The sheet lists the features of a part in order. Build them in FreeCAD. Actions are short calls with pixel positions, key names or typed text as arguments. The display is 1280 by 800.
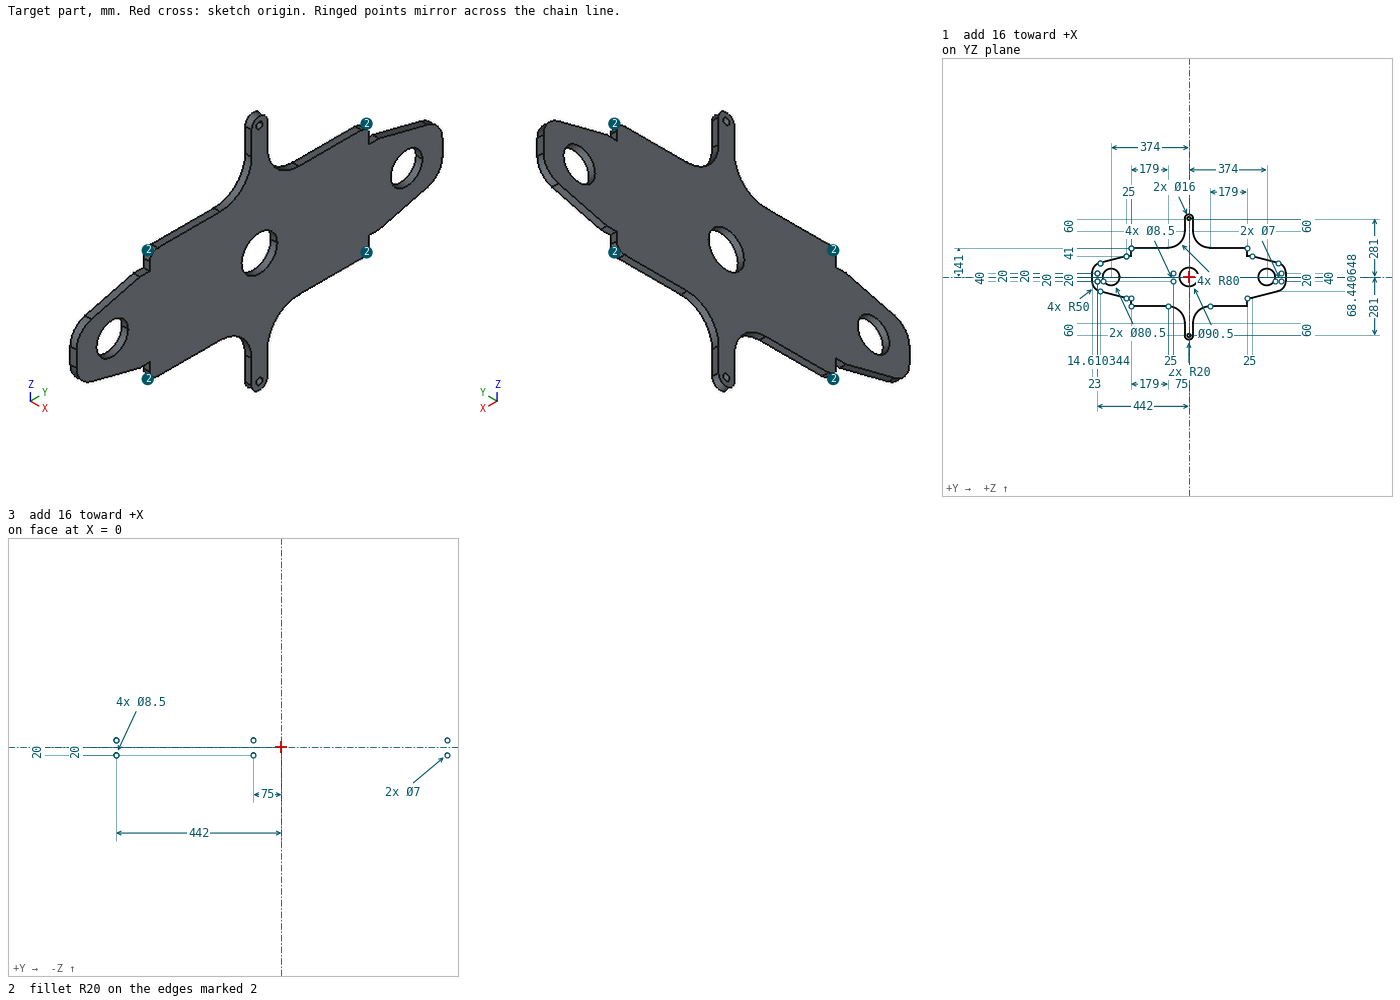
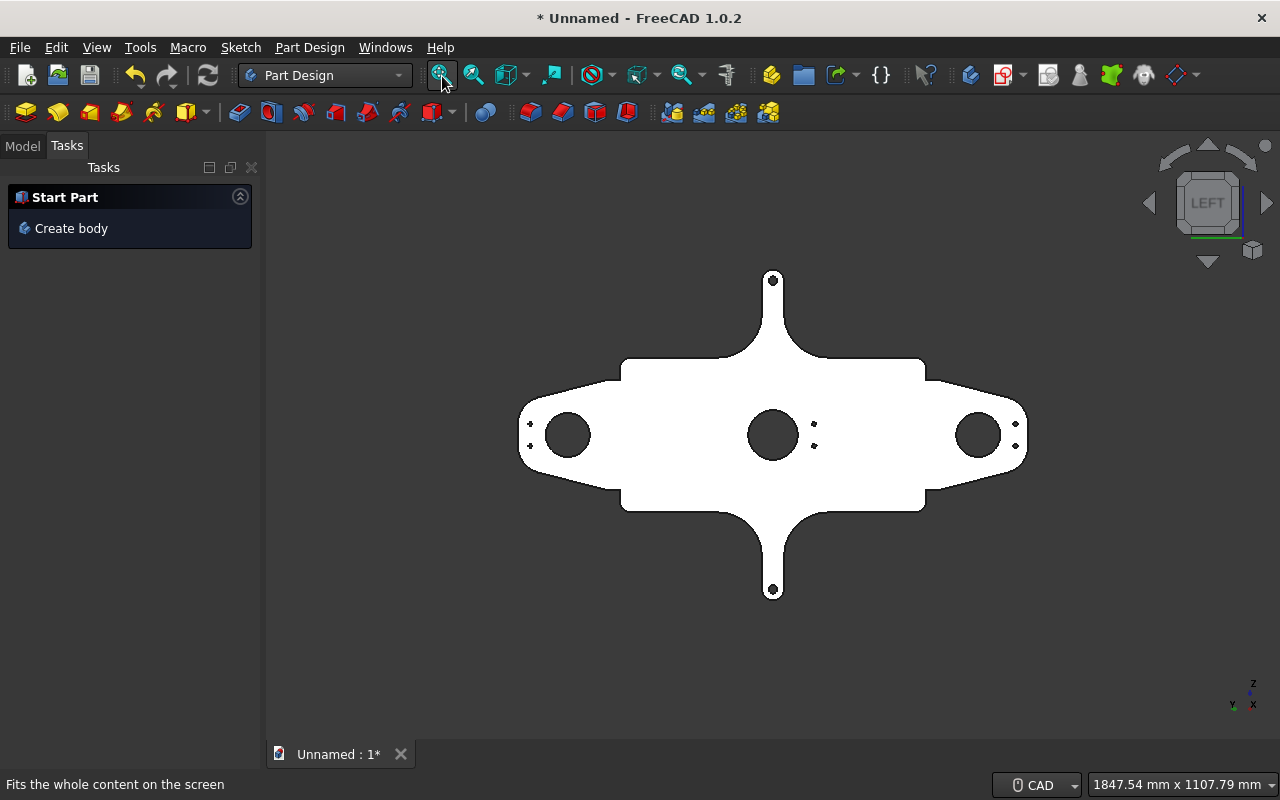
click(700, 434)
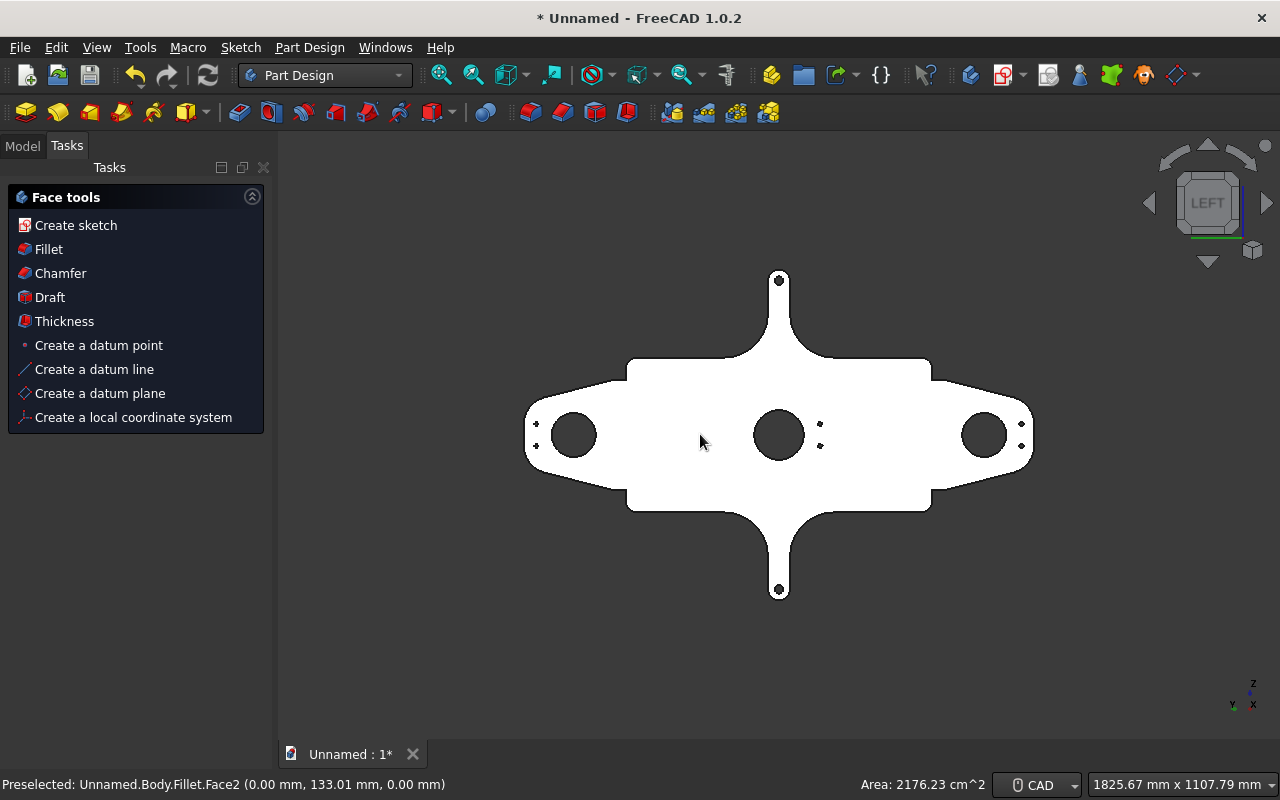
click(1004, 76)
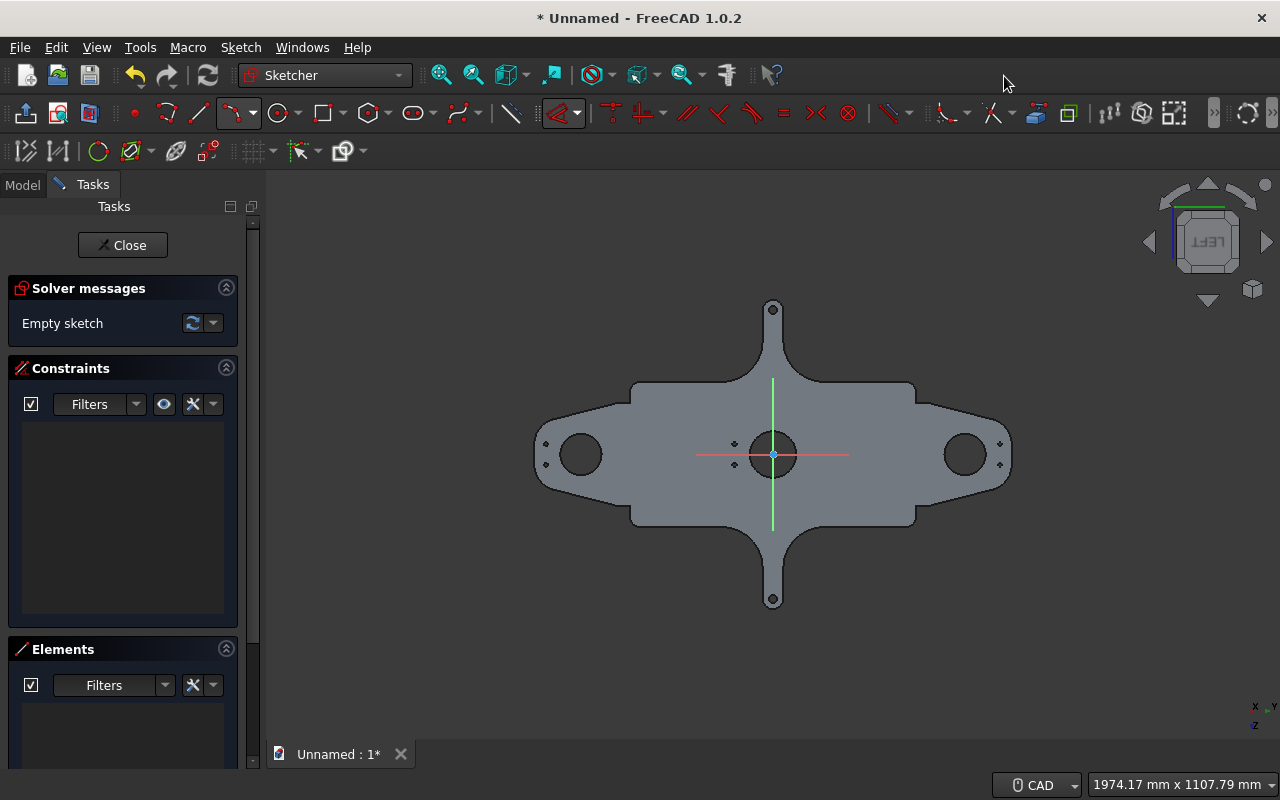
key(g)
key(c)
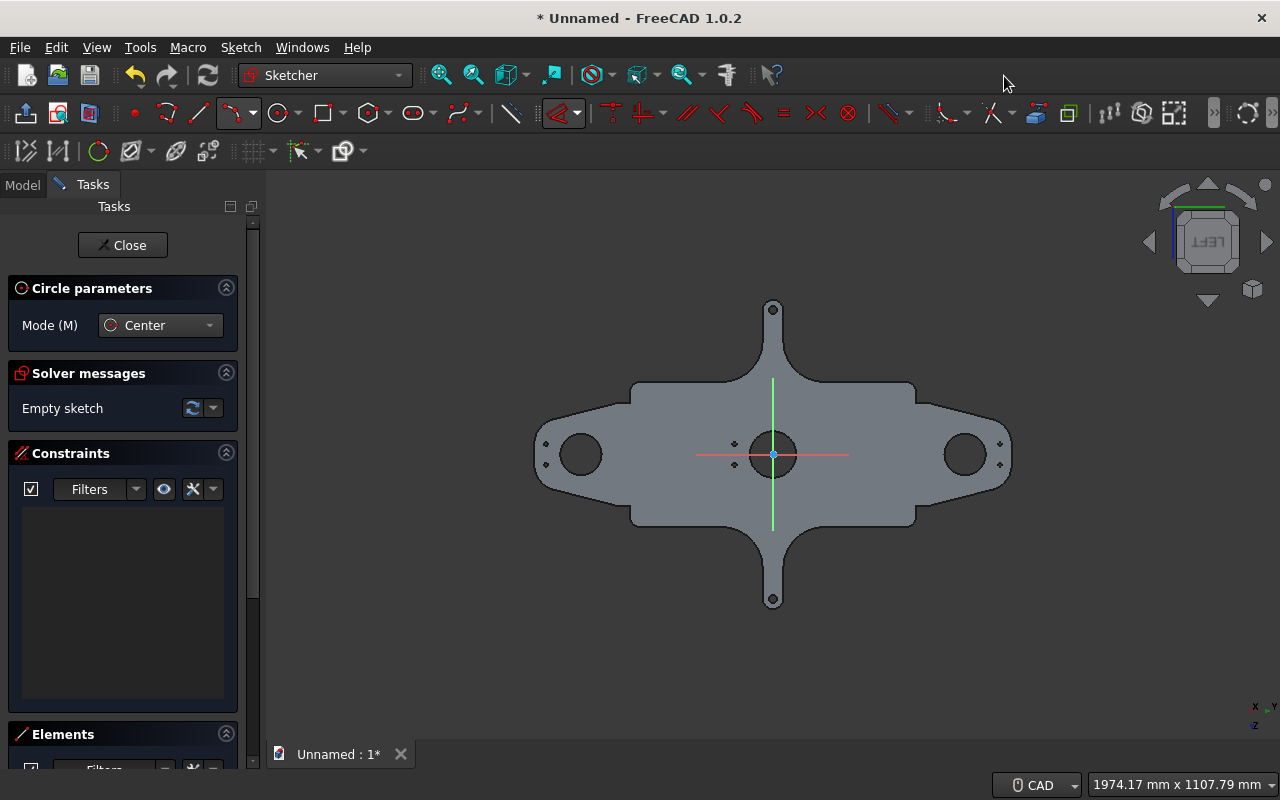
scroll(546, 465, up, 12)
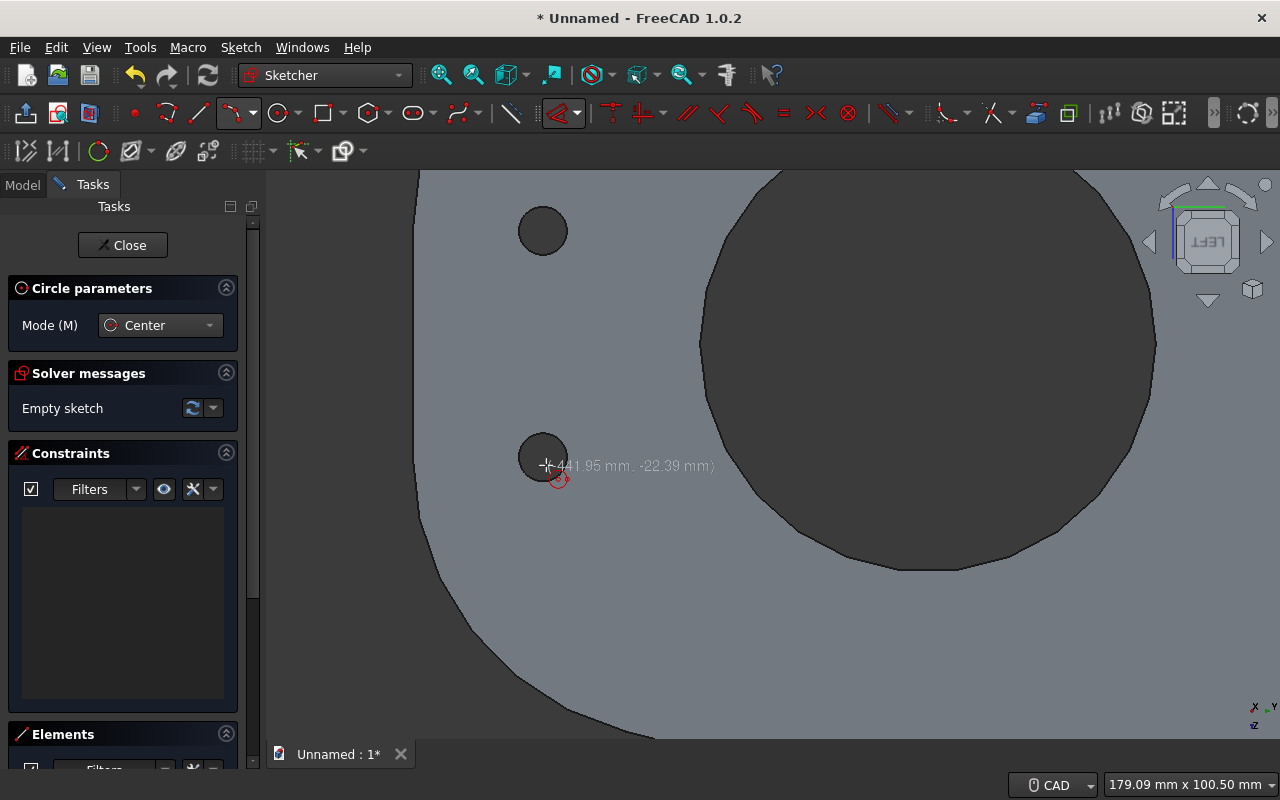
scroll(413, 468, down, 11)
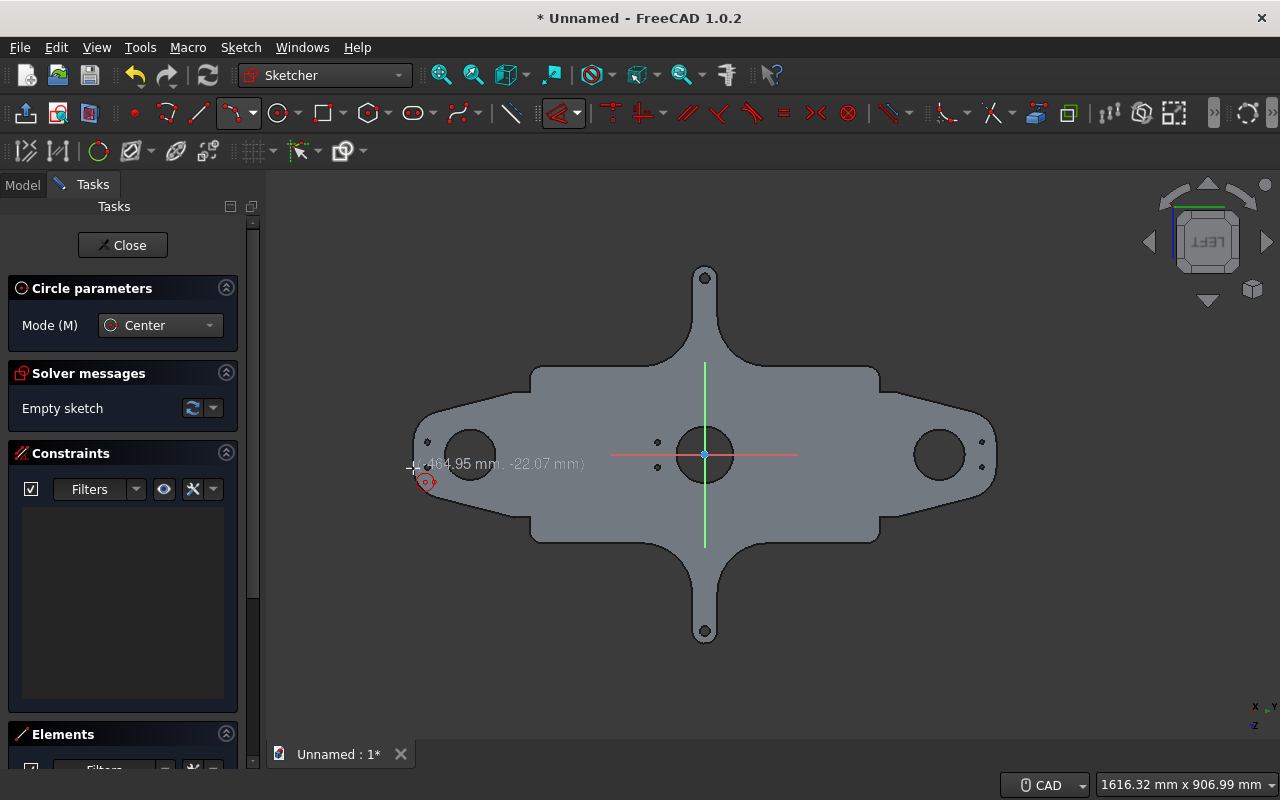
scroll(428, 467, up, 2)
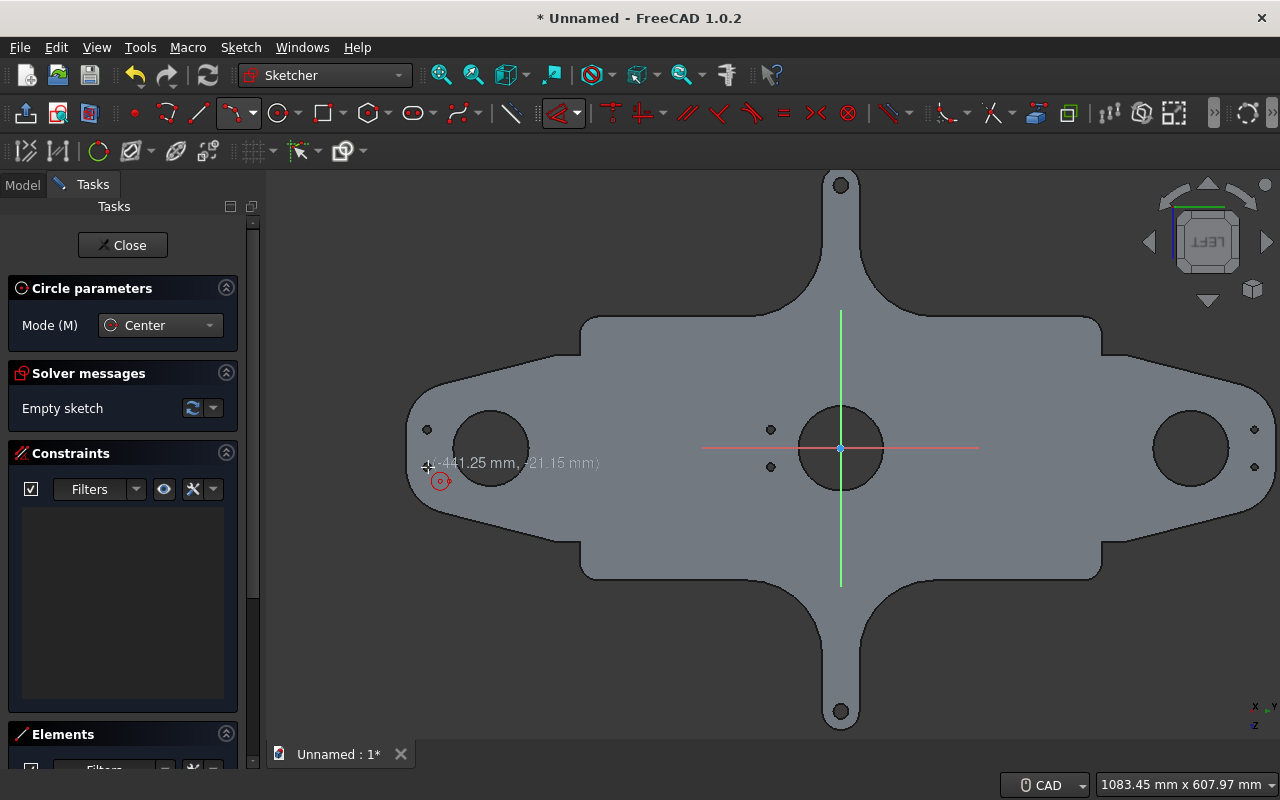
click(427, 467)
move(430, 464)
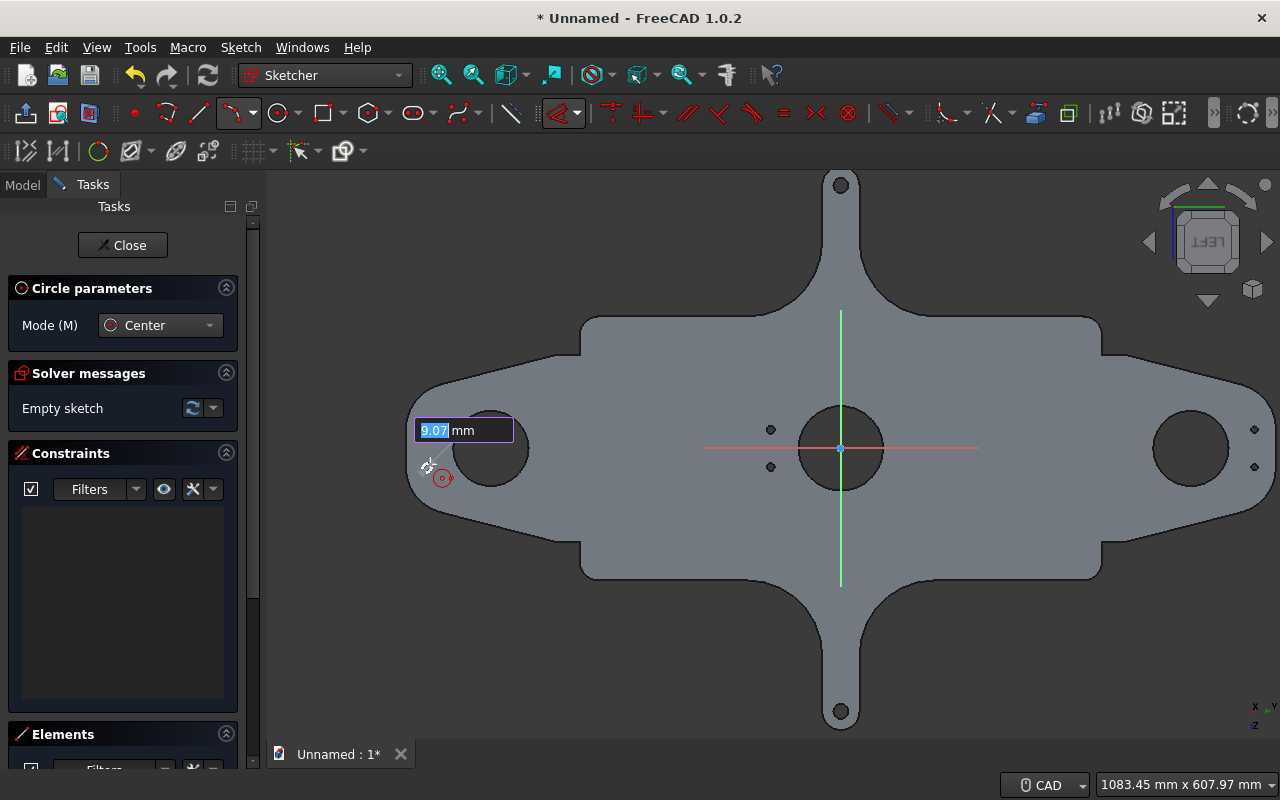
text(8.5)
key(Return)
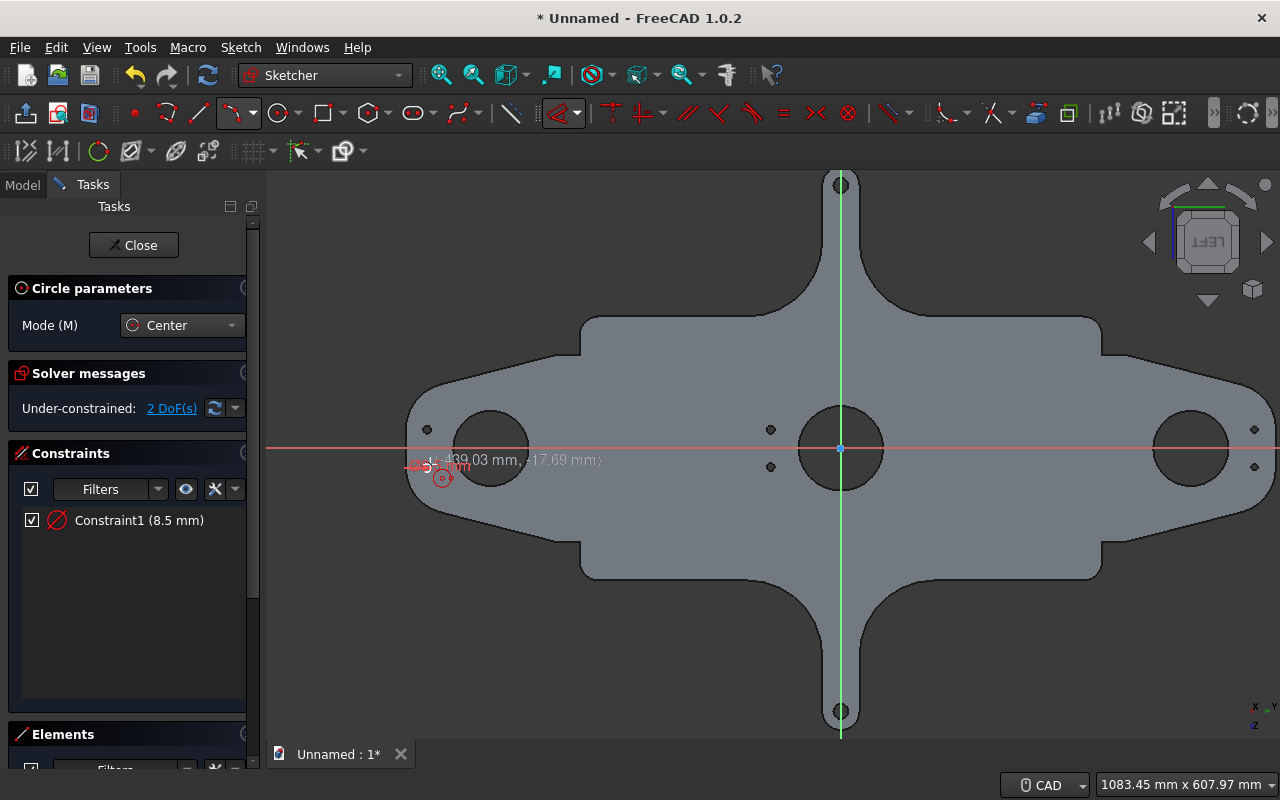
scroll(427, 430, up, 9)